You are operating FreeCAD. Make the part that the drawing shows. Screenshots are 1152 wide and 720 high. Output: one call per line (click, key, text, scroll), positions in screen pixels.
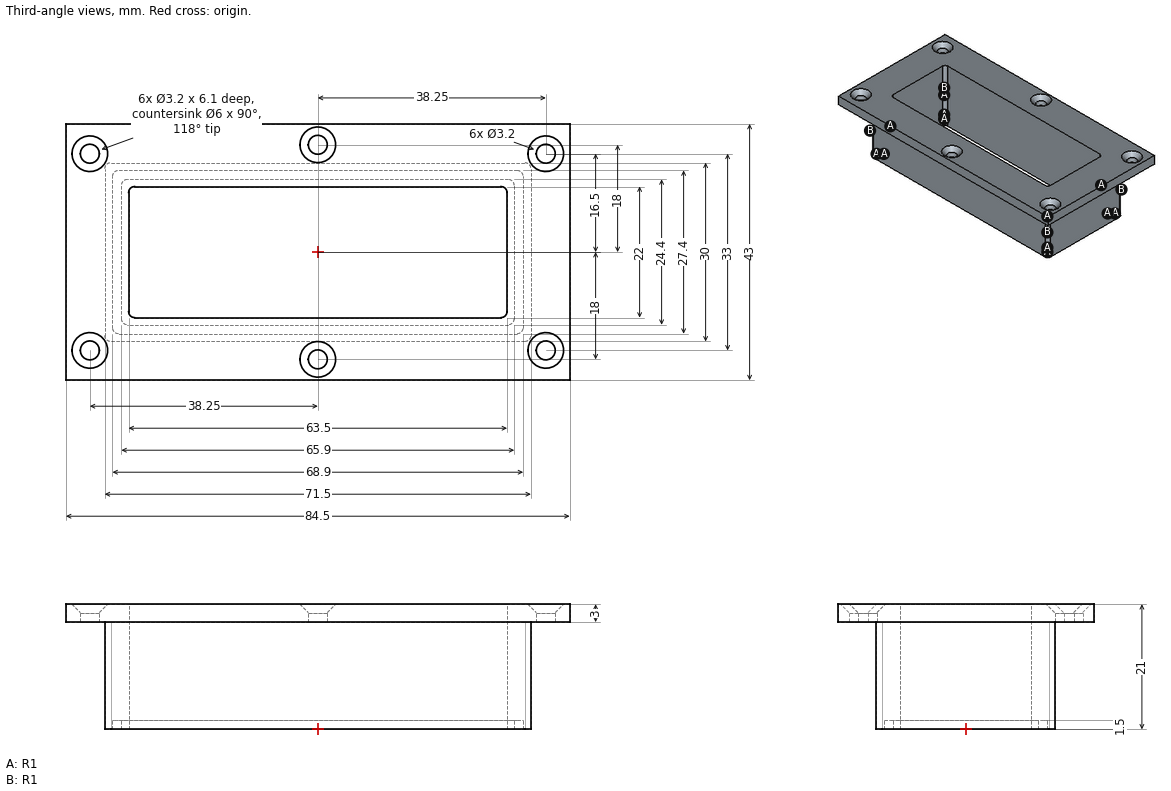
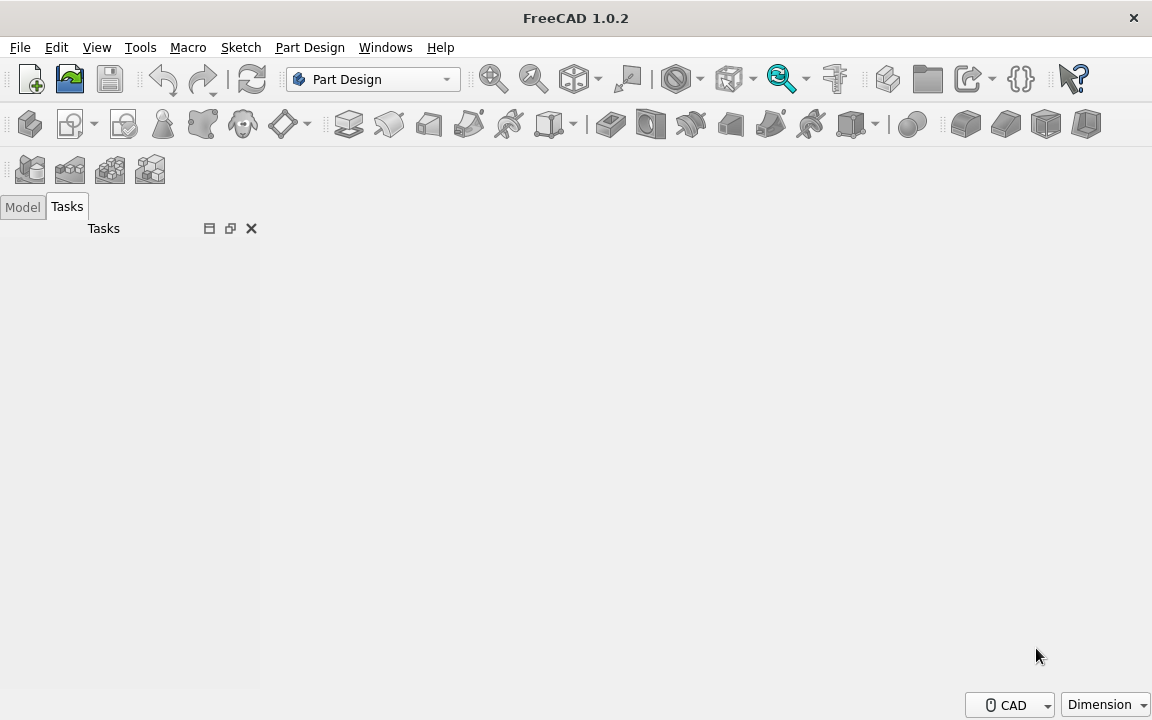
key(ctrl+n)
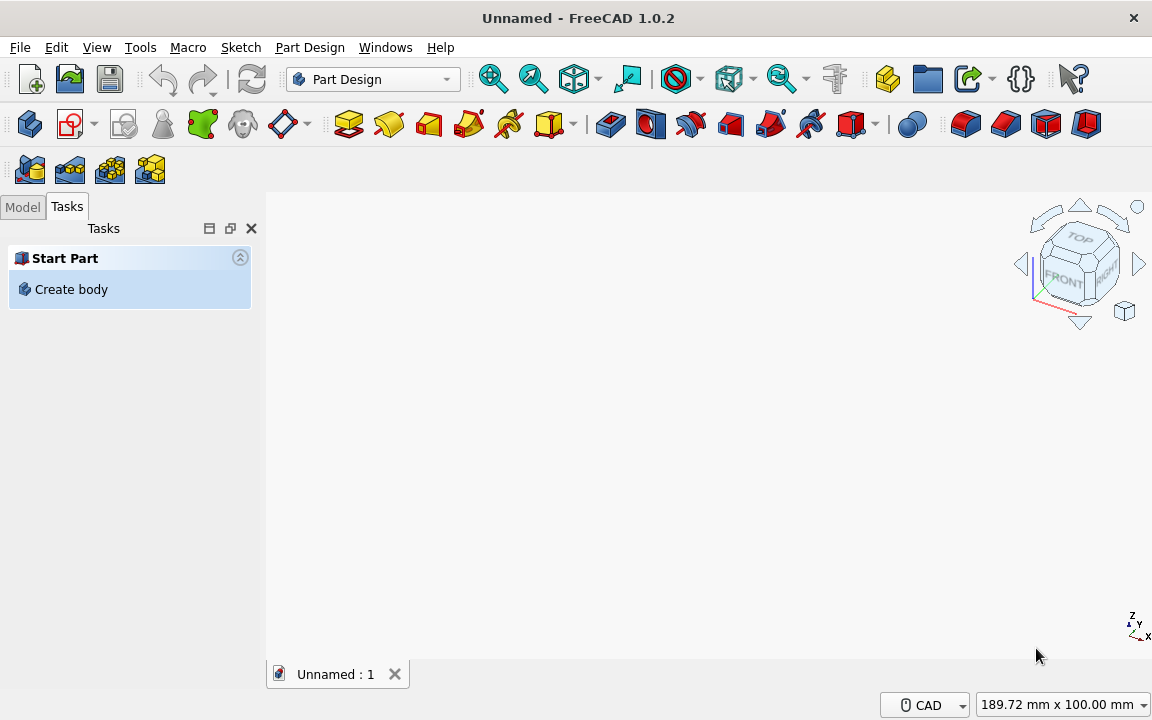
click(70, 124)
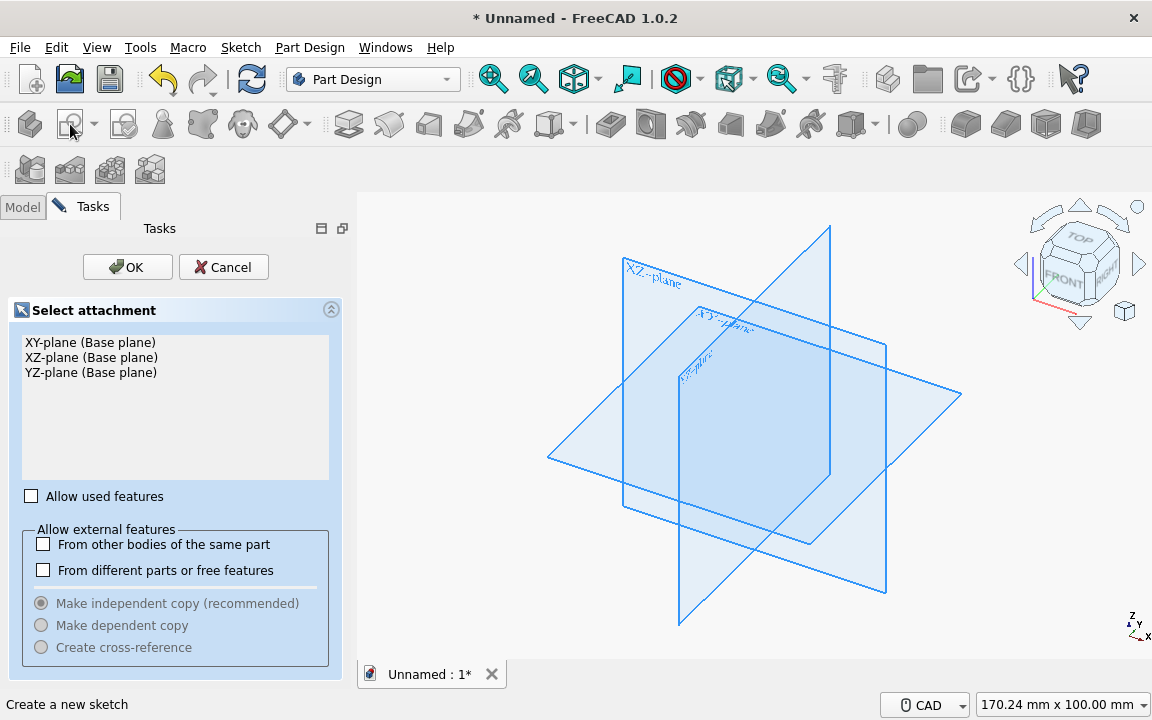
click(82, 342)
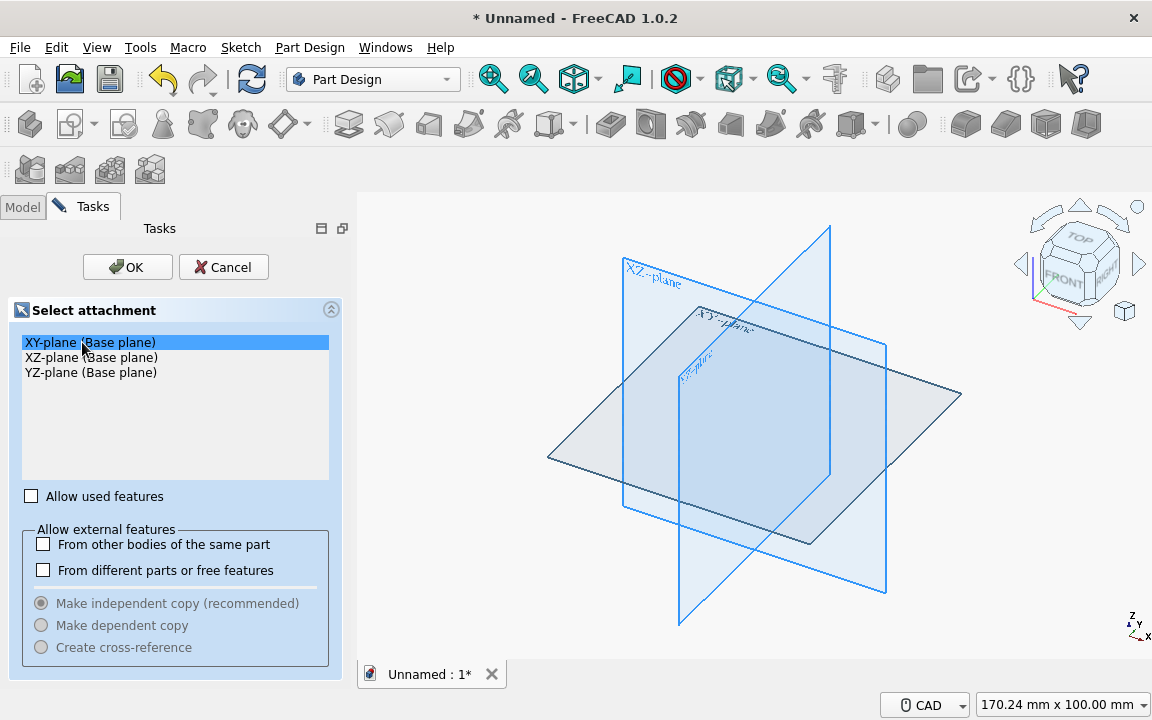
click(128, 267)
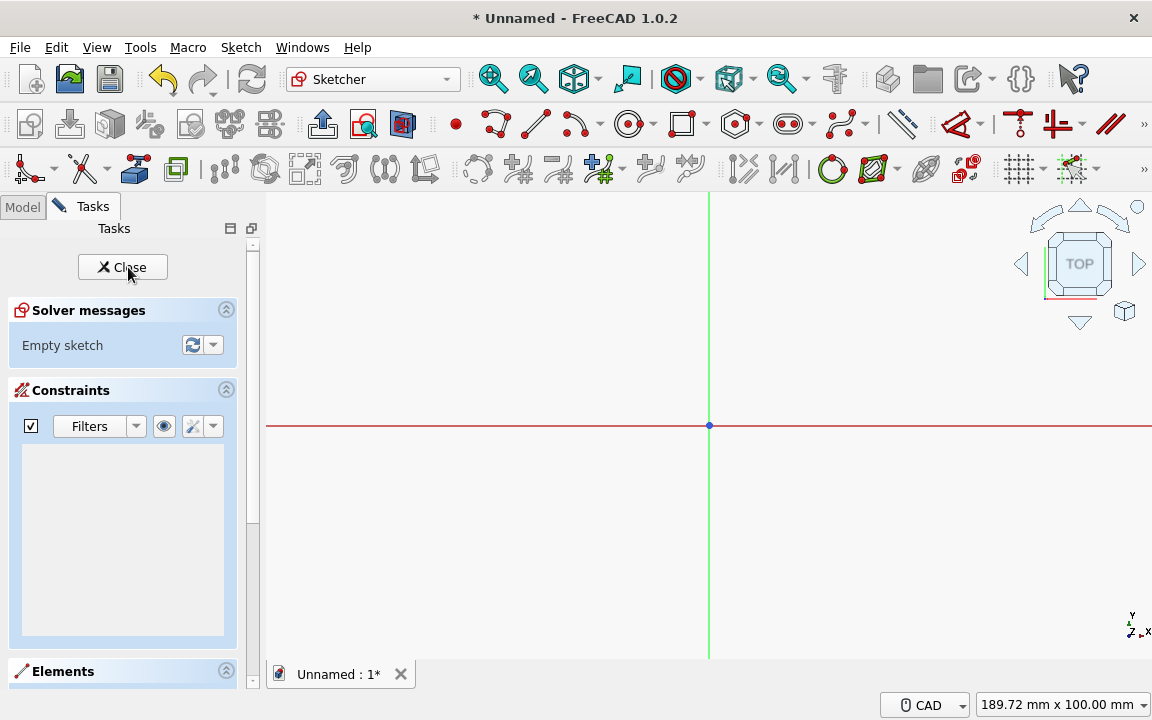
scroll(848, 425, up, 2)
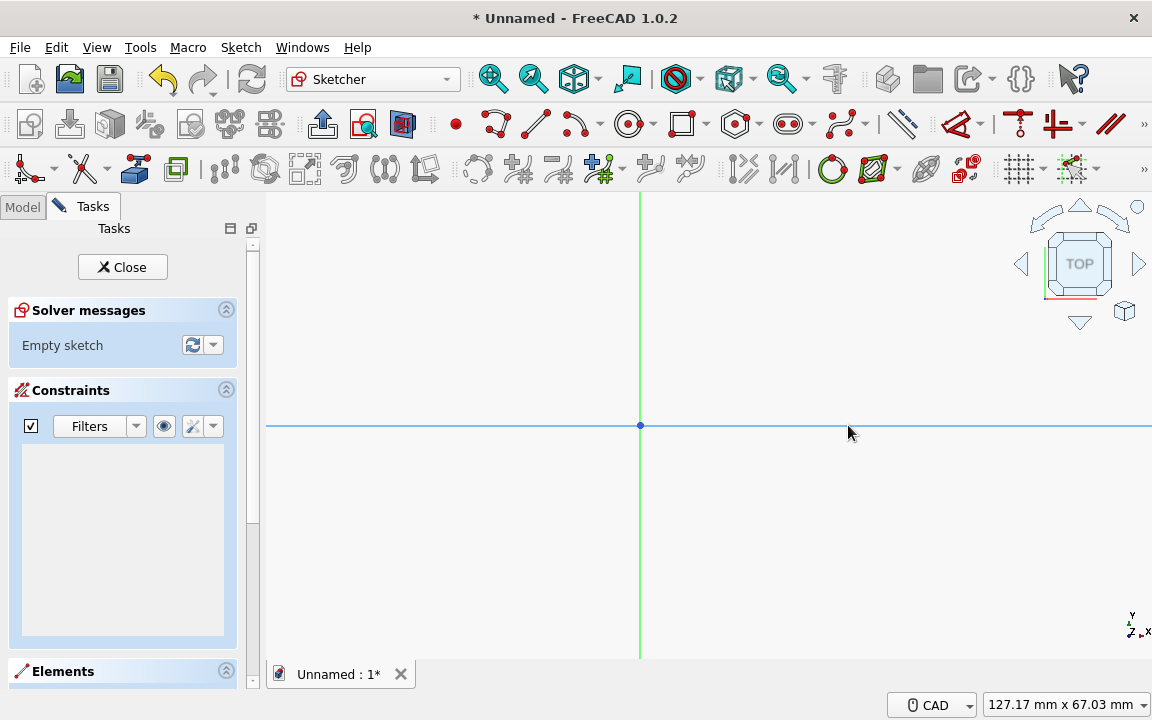
key(g)
key(v)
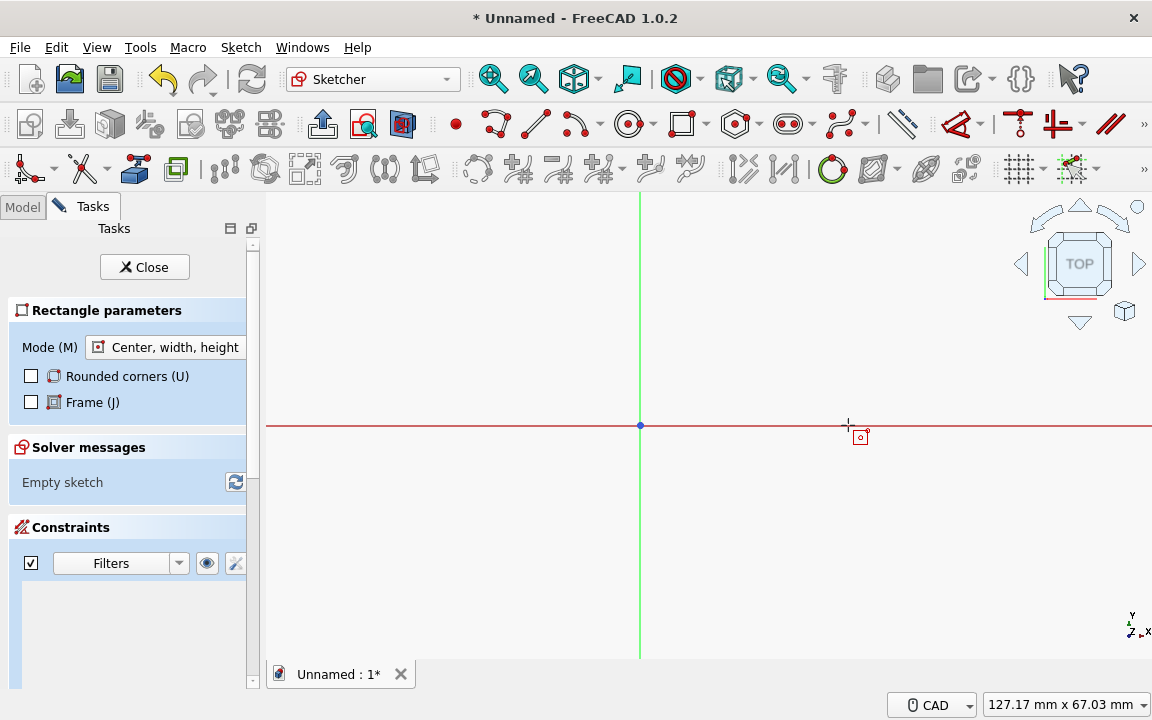
click(640, 426)
click(889, 321)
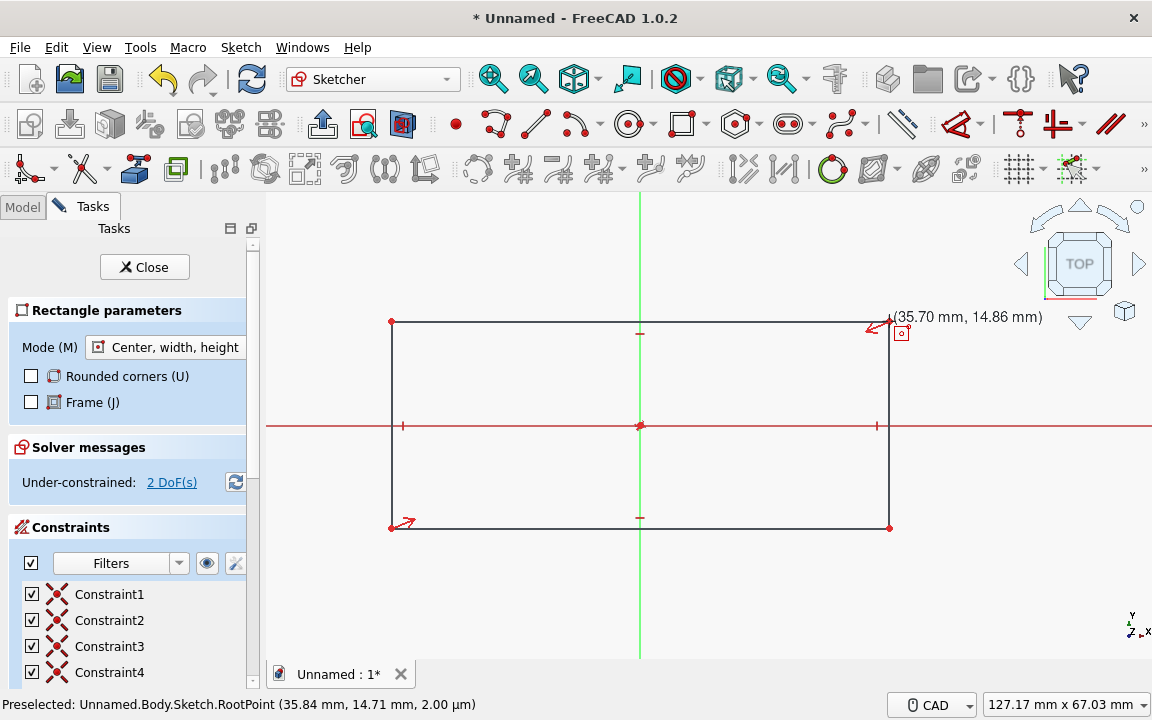
click(640, 426)
click(862, 349)
key(Escape)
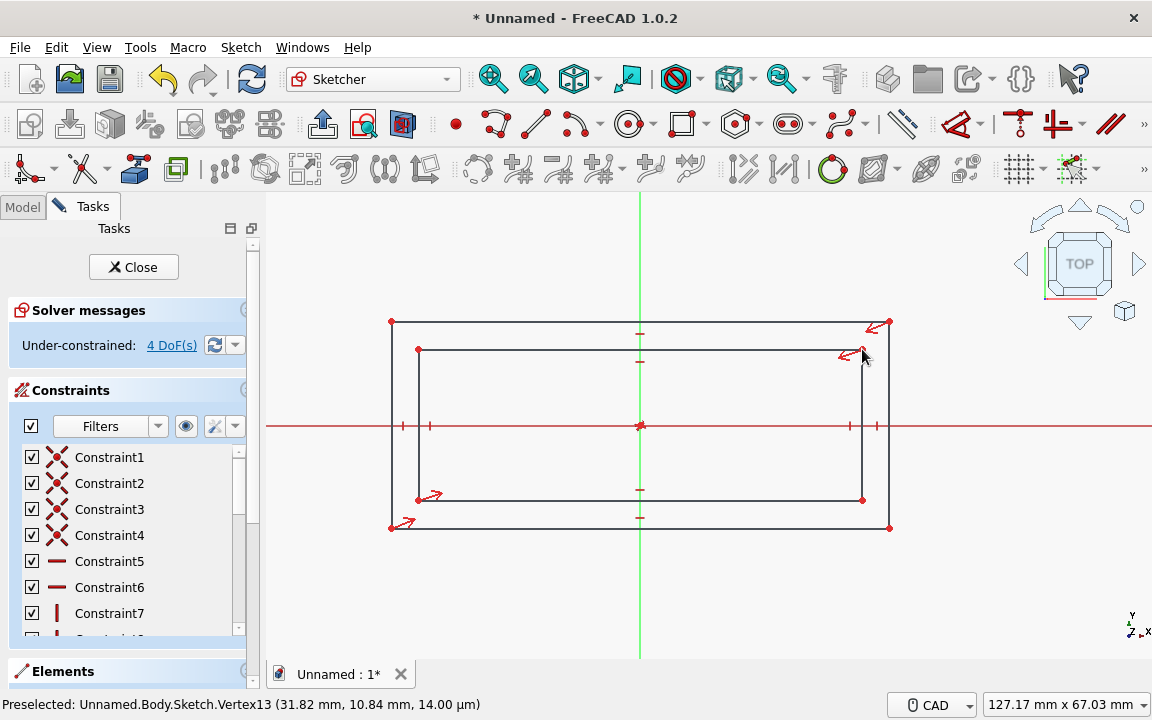
click(956, 124)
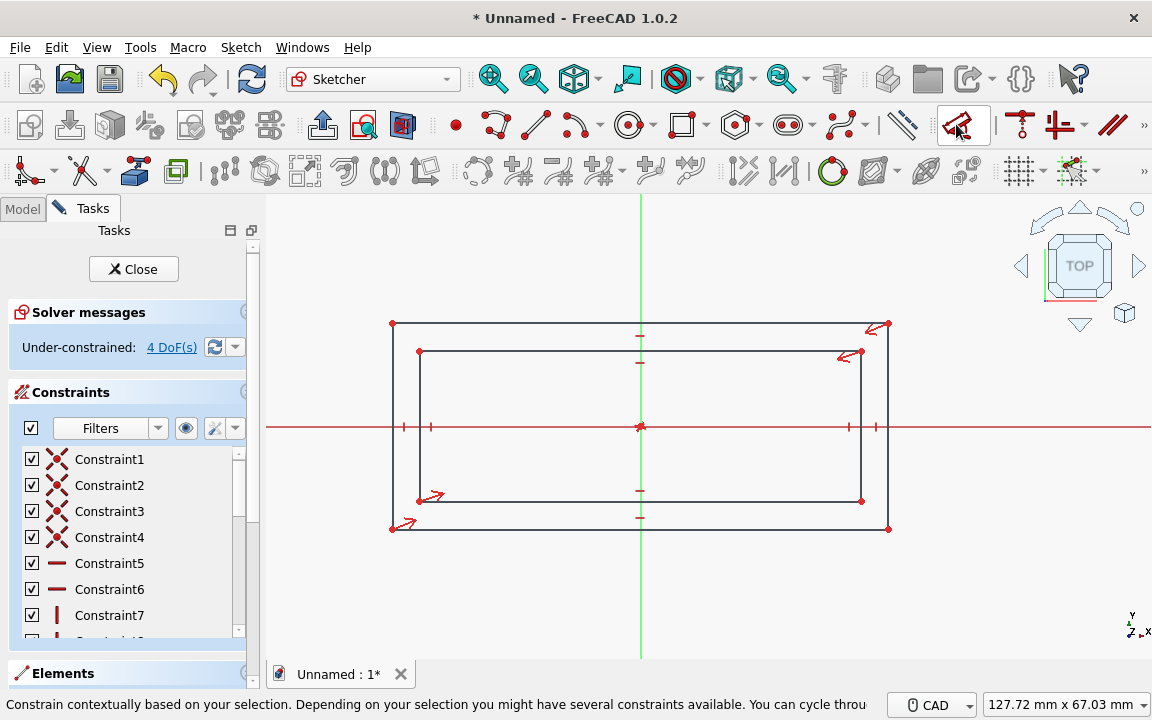
click(888, 468)
click(922, 379)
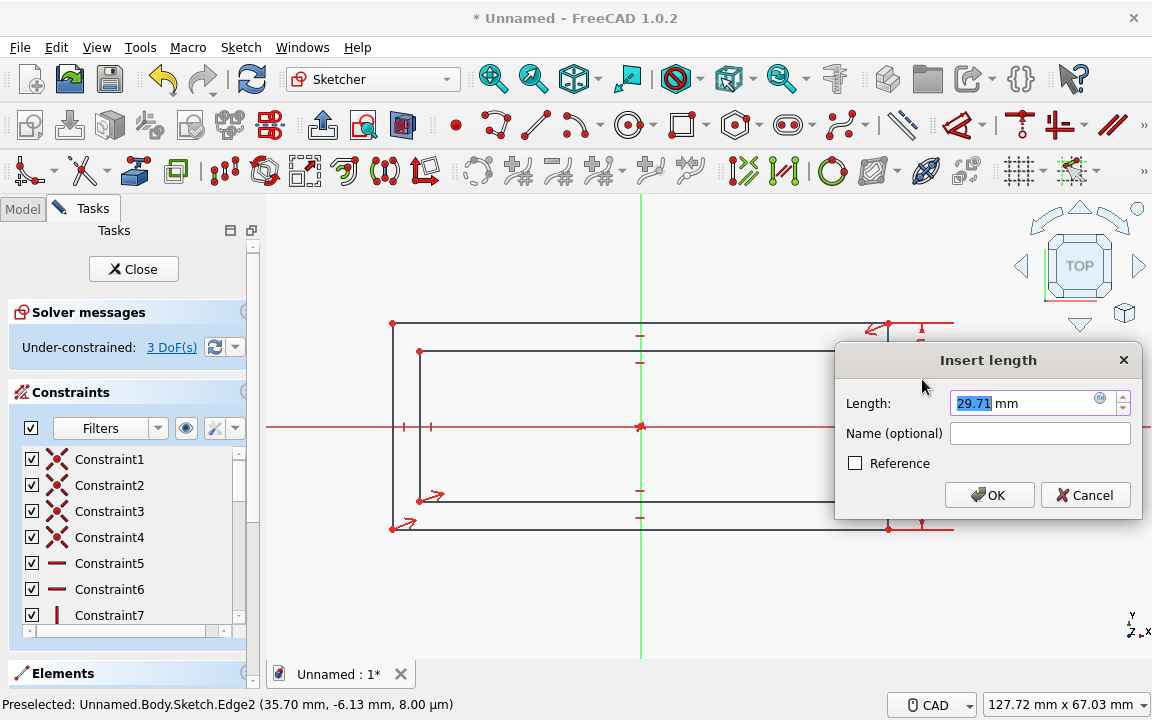
text(30)
key(Return)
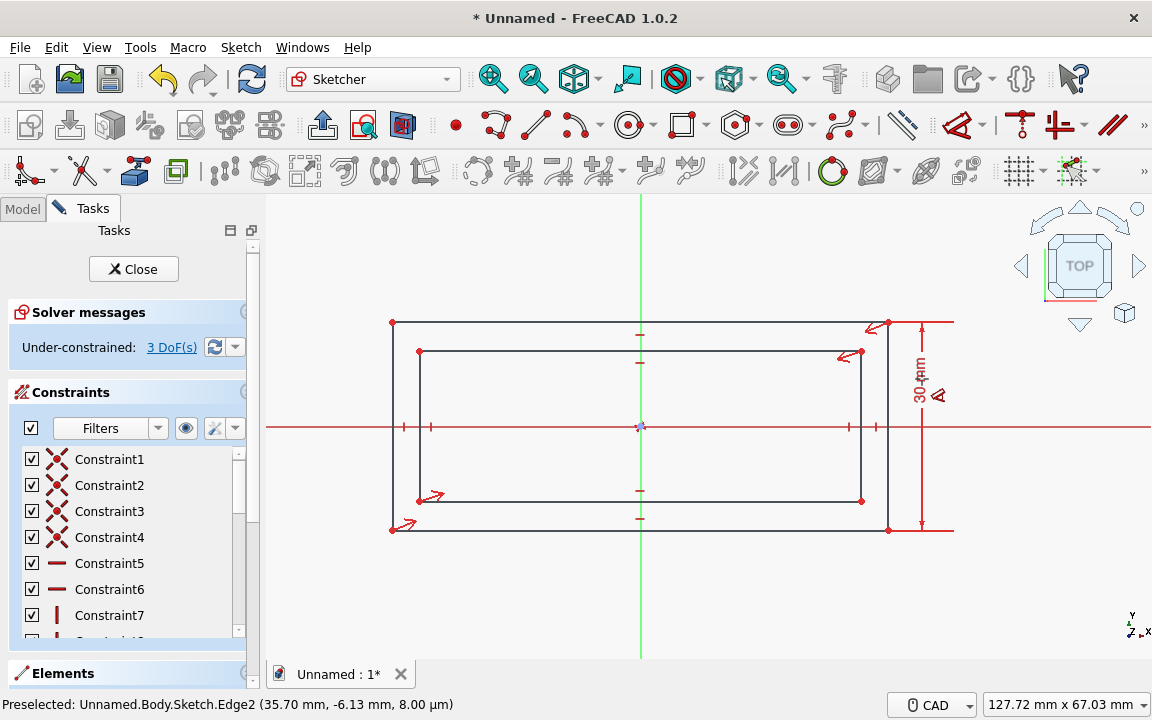
click(861, 457)
click(827, 392)